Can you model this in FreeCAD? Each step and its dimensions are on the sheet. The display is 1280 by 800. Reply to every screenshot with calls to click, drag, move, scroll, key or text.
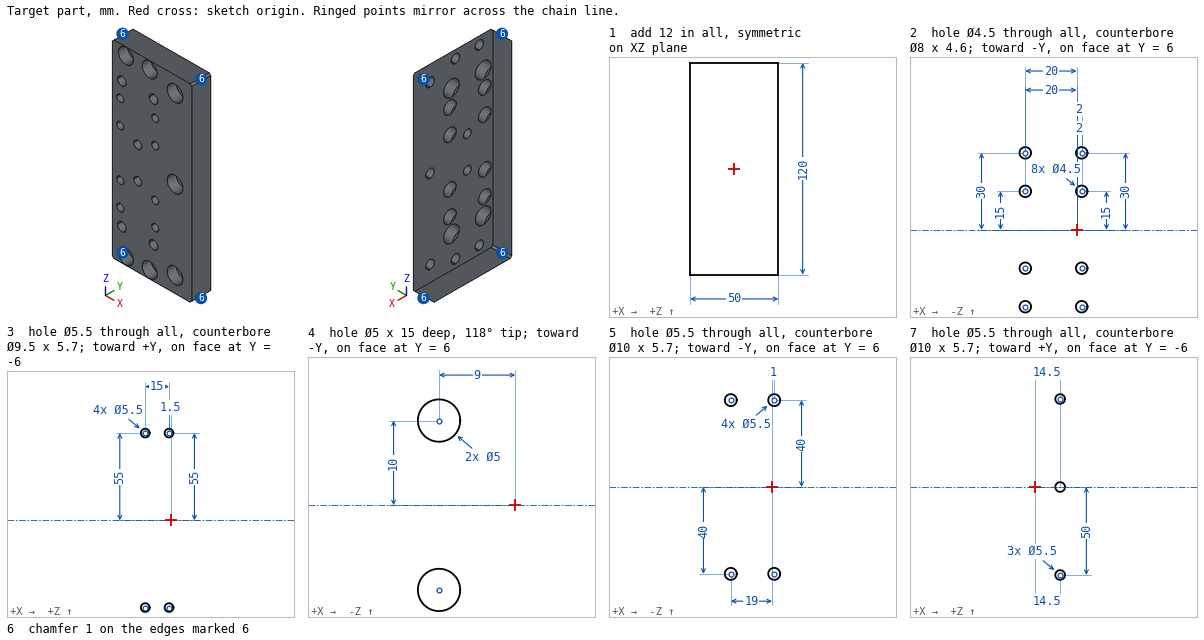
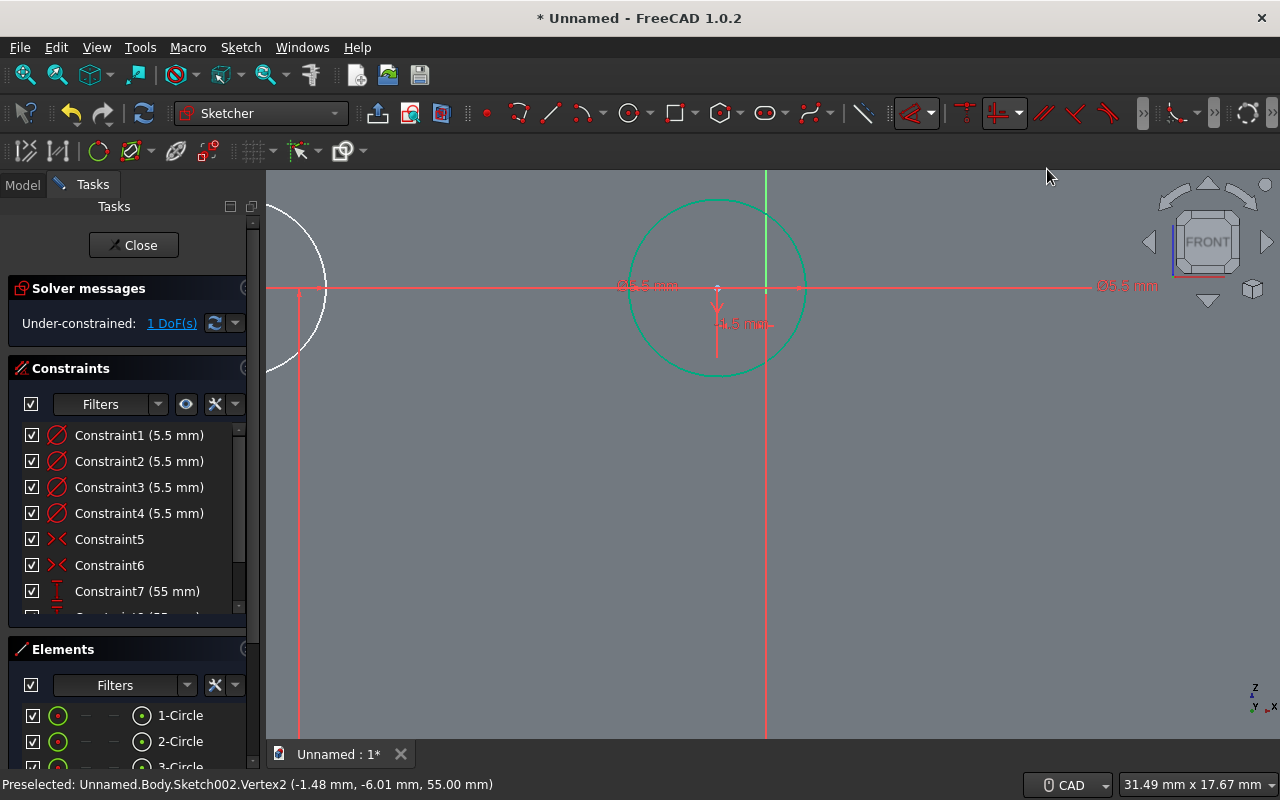
scroll(727, 294, down, 12)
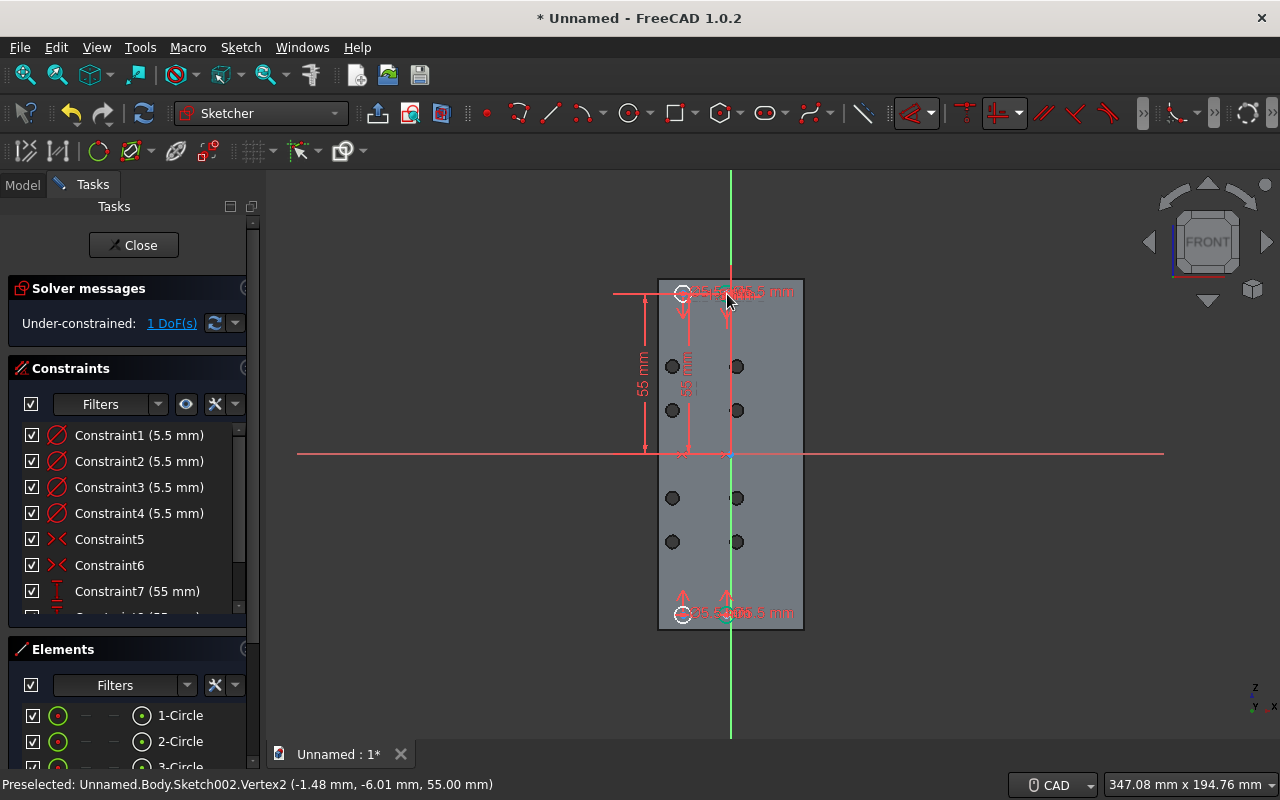
click(683, 294)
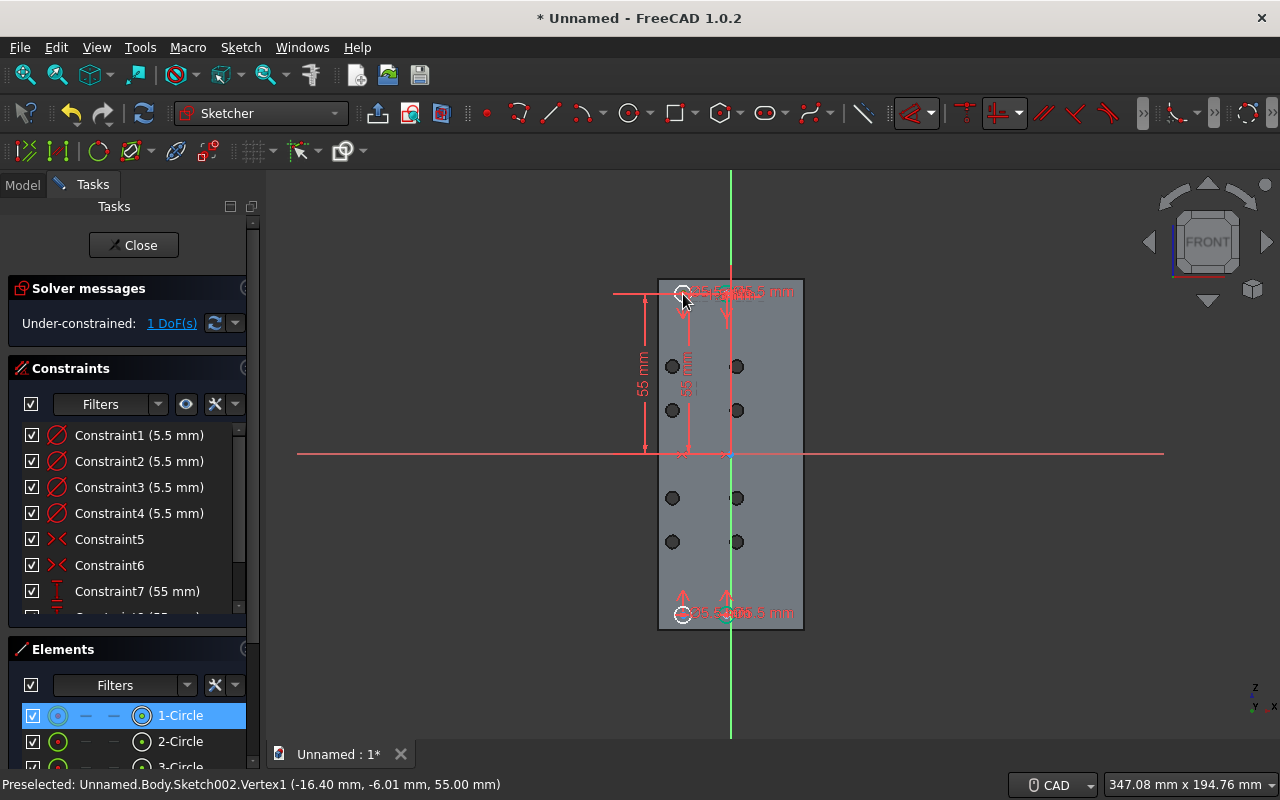
click(727, 294)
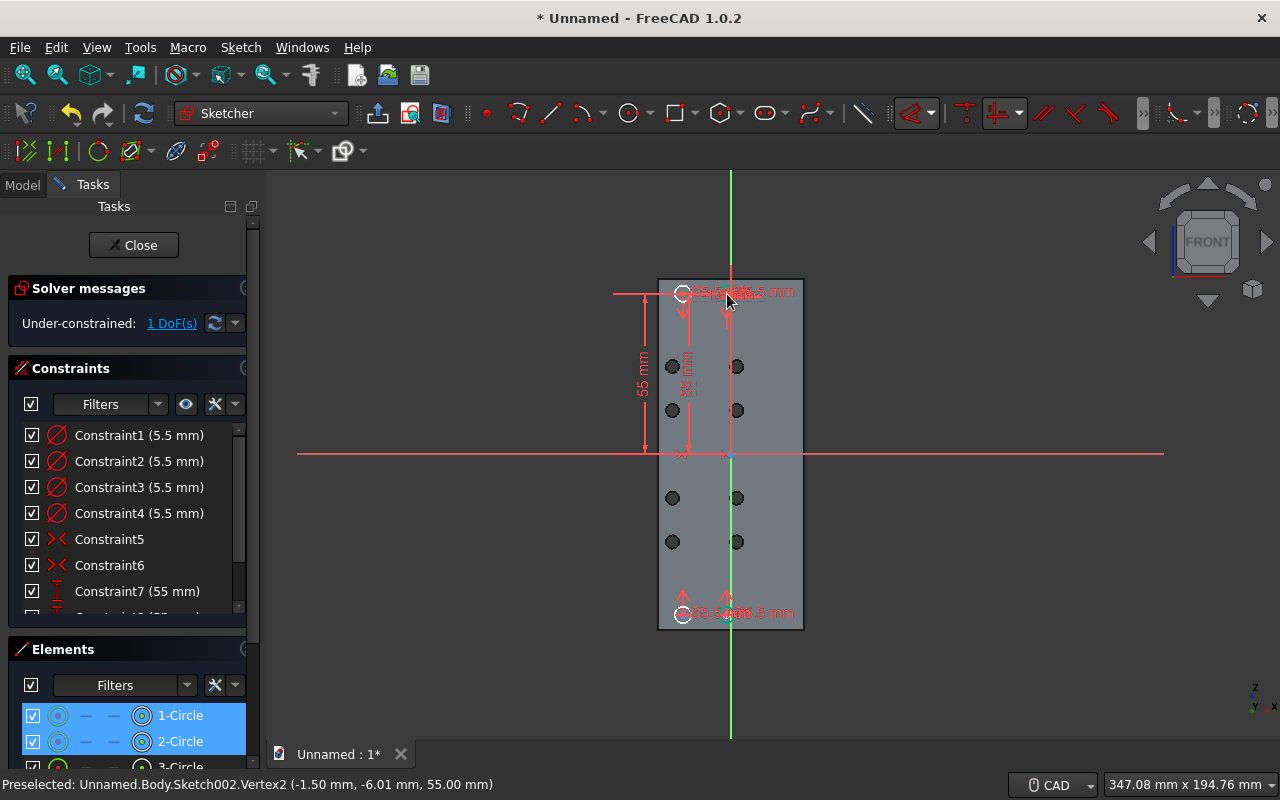
click(934, 114)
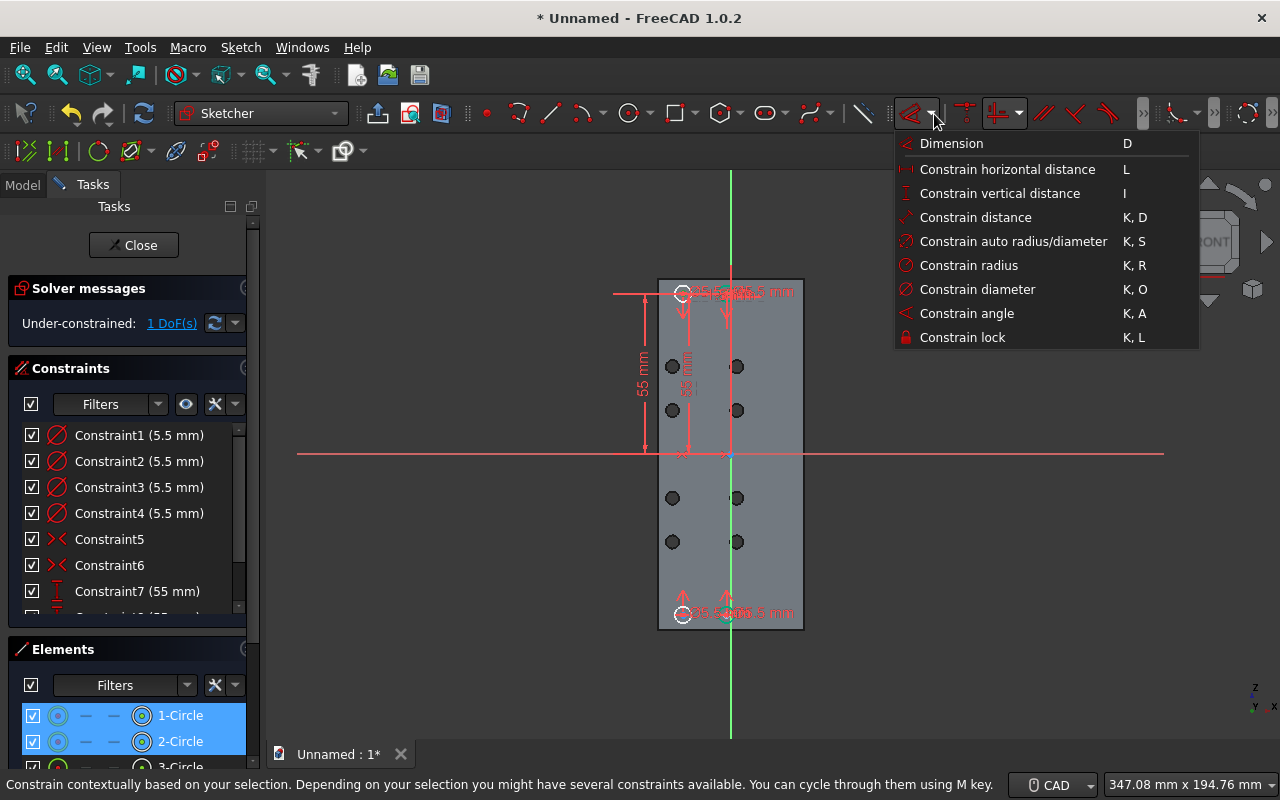
click(1047, 169)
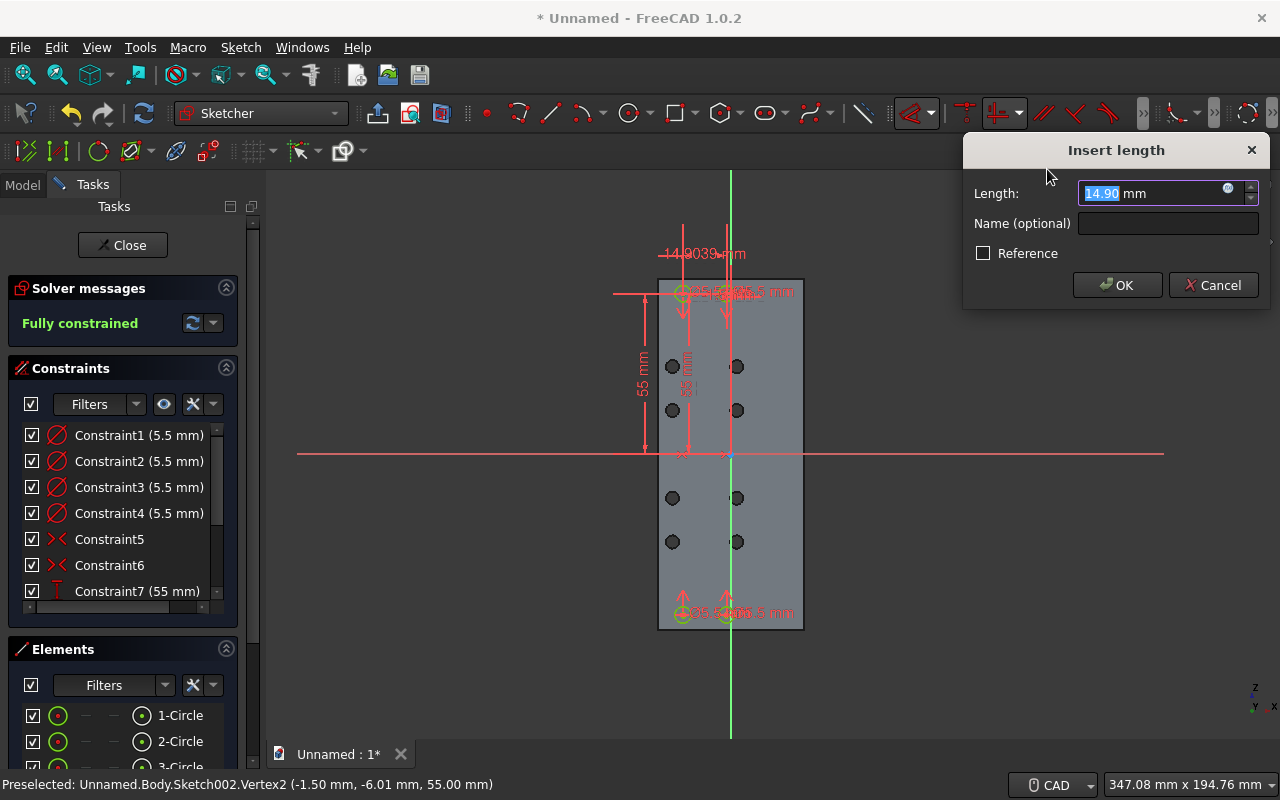
text(15)
key(Return)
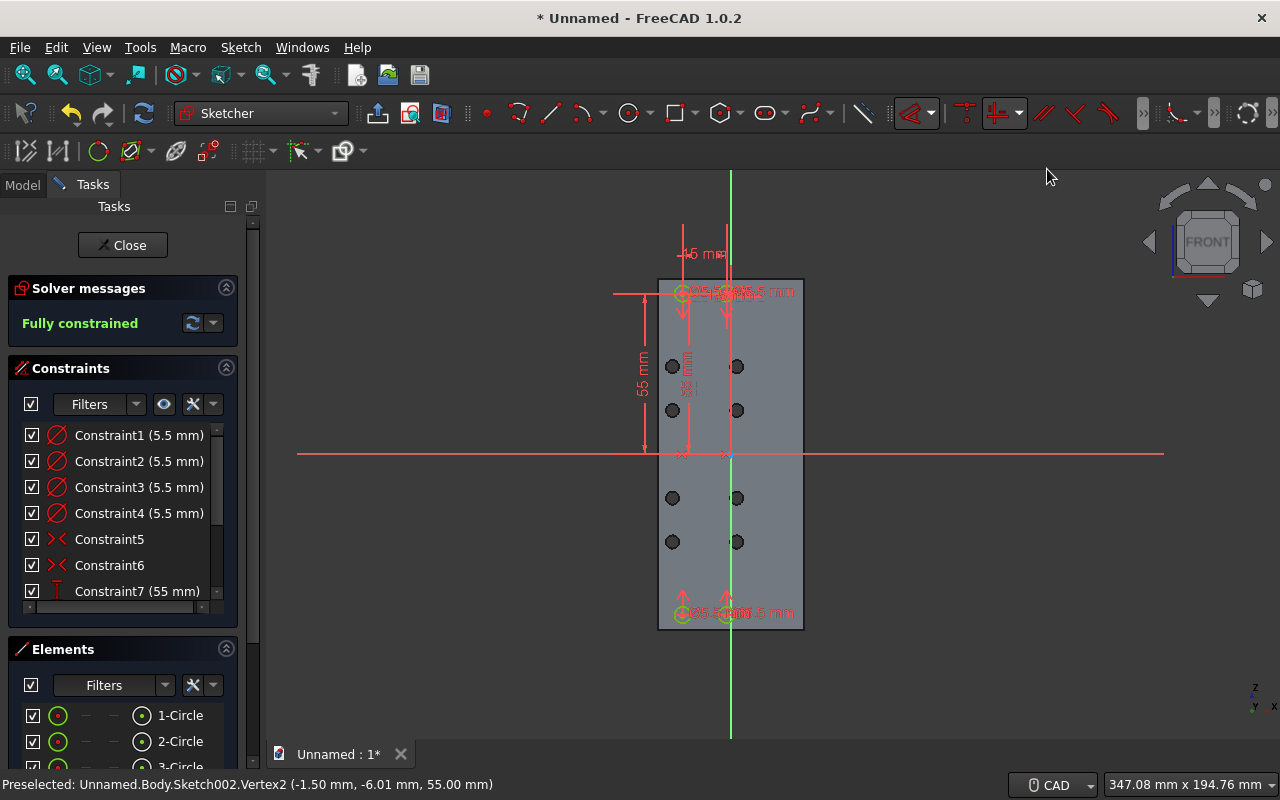
click(123, 245)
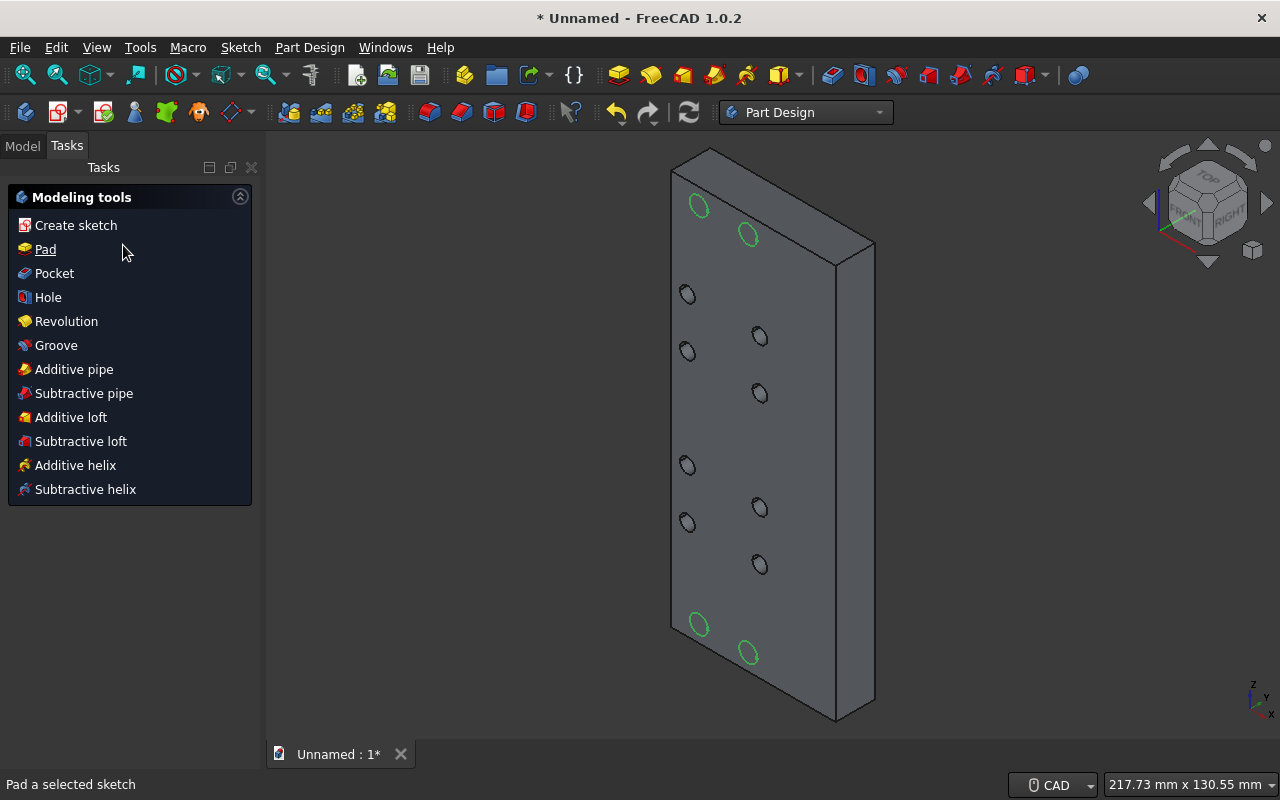
click(866, 76)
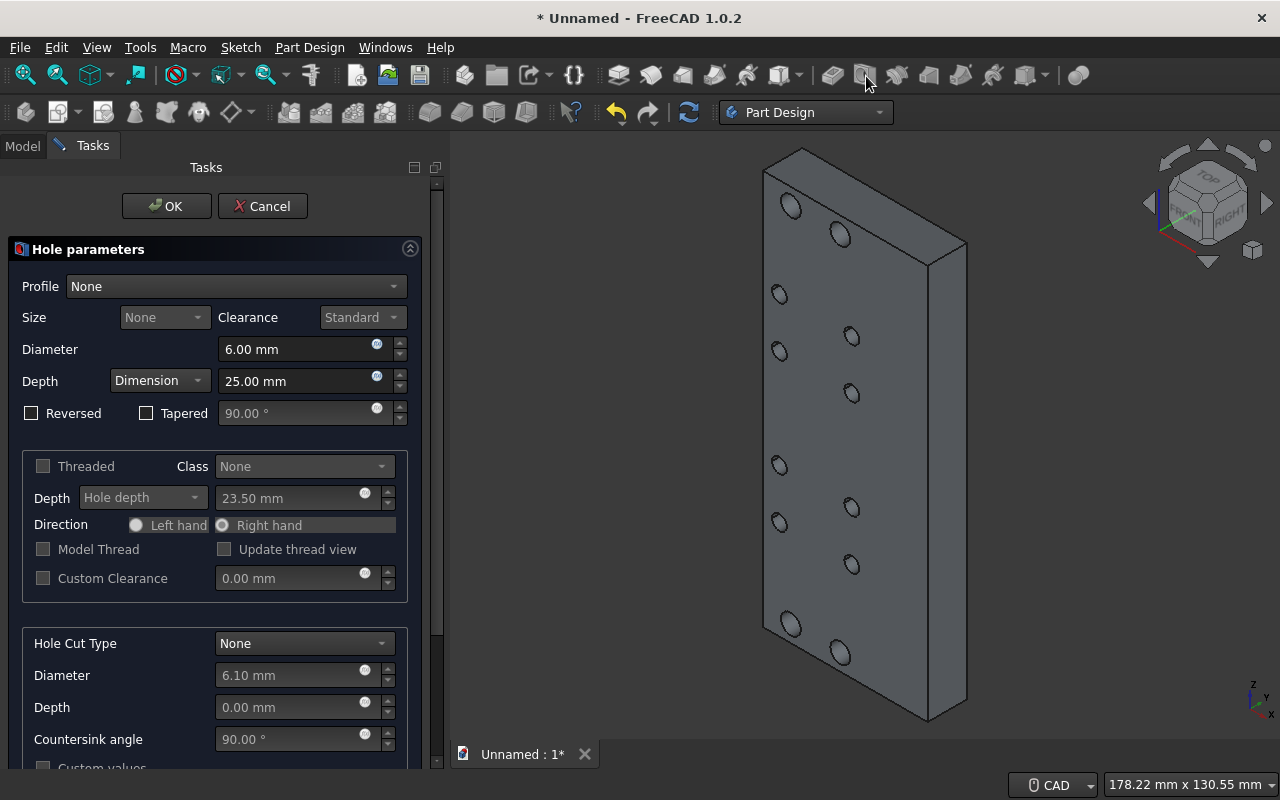
triple_click(305, 349)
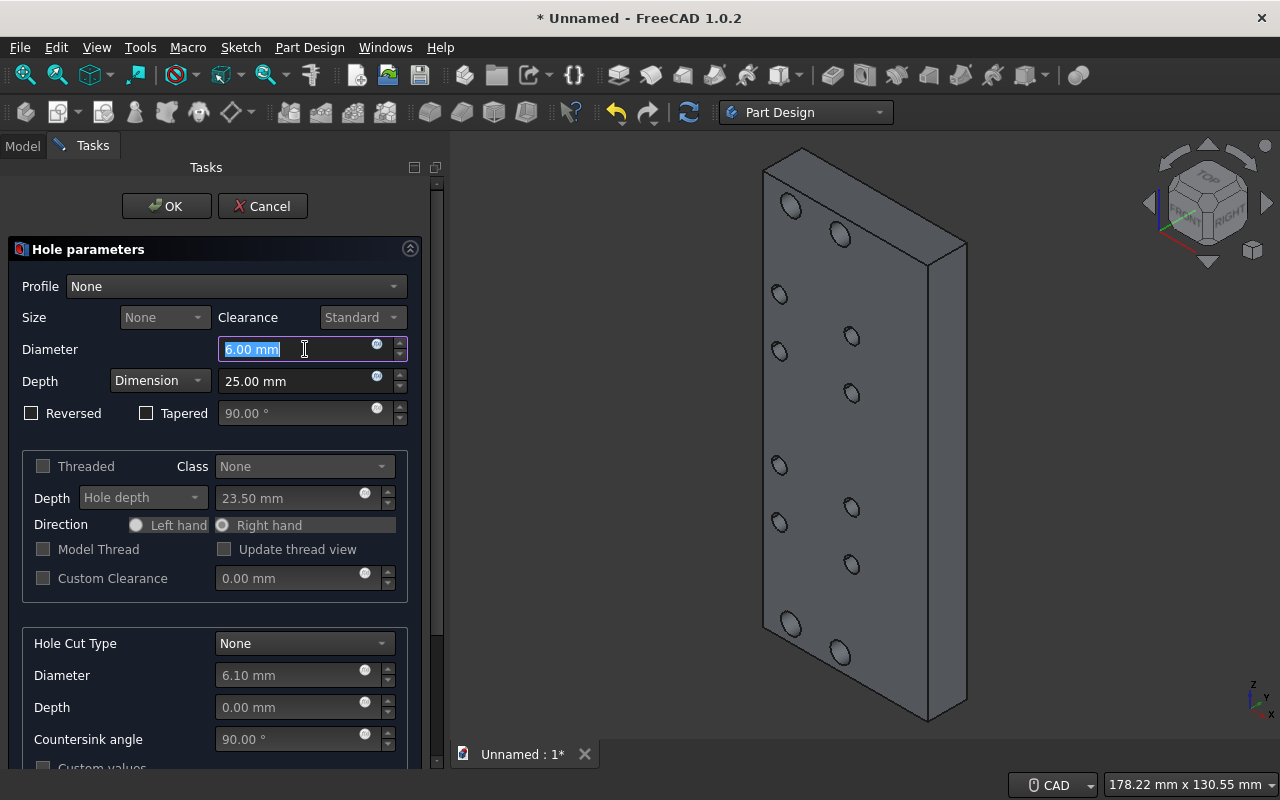
text(5.5)
key(Tab)